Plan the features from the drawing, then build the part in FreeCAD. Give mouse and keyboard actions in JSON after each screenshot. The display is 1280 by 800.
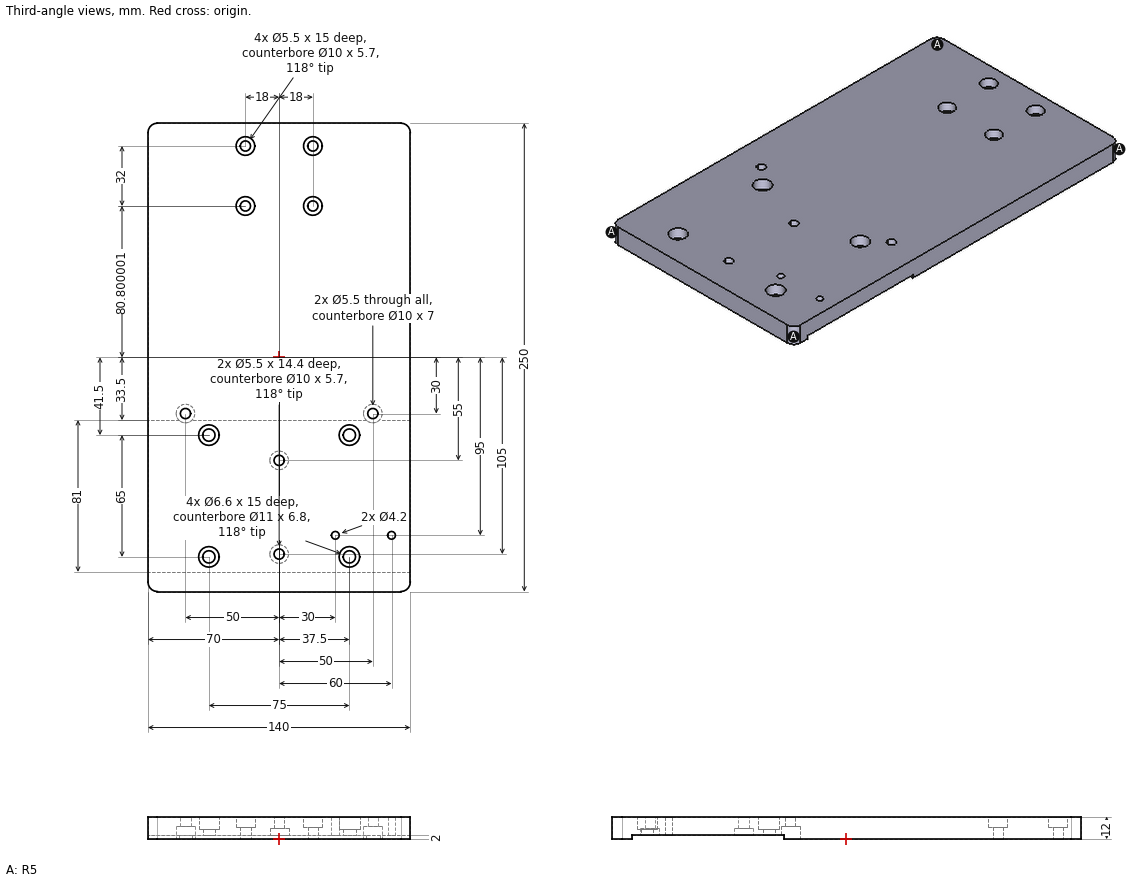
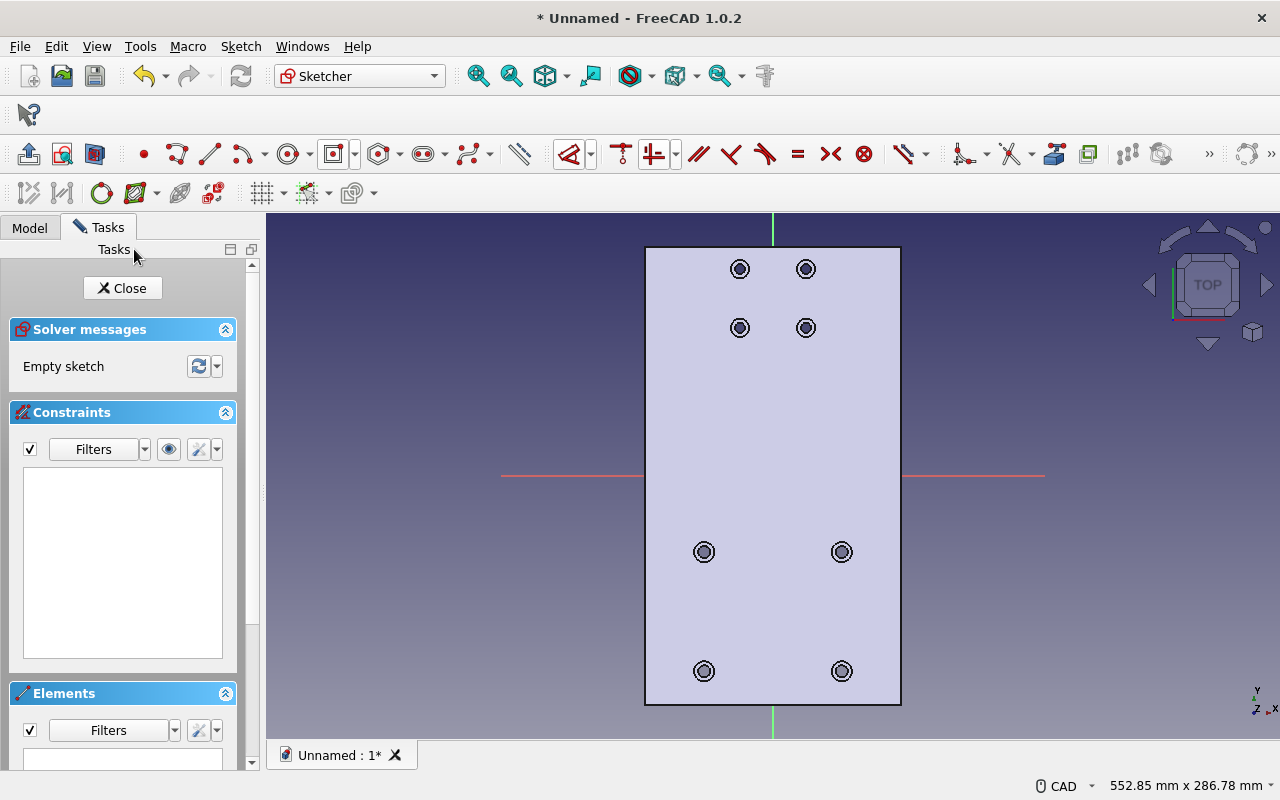
{"action": "left_click", "coordinate": [95, 154]}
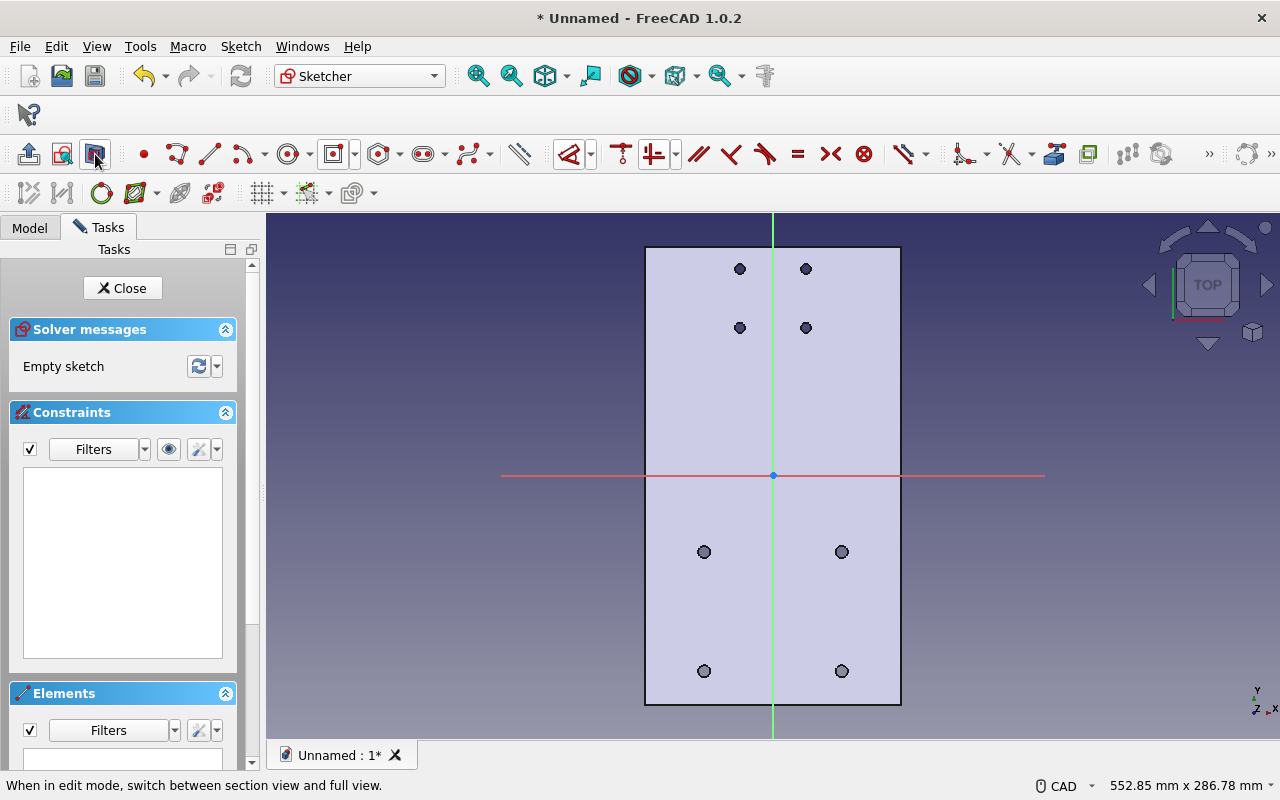
{"action": "scroll", "coordinate": [856, 695], "scroll_direction": "up", "scroll_amount": 3}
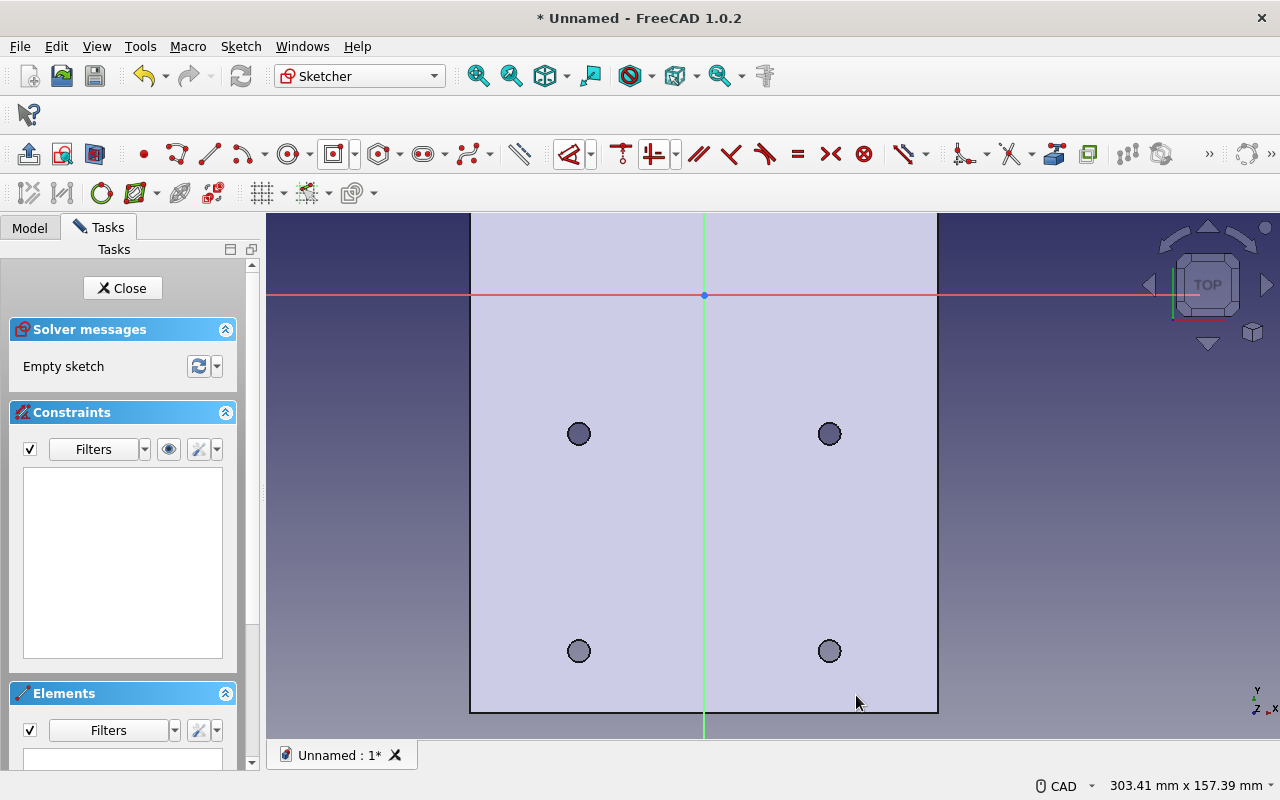
{"action": "left_click", "coordinate": [288, 154]}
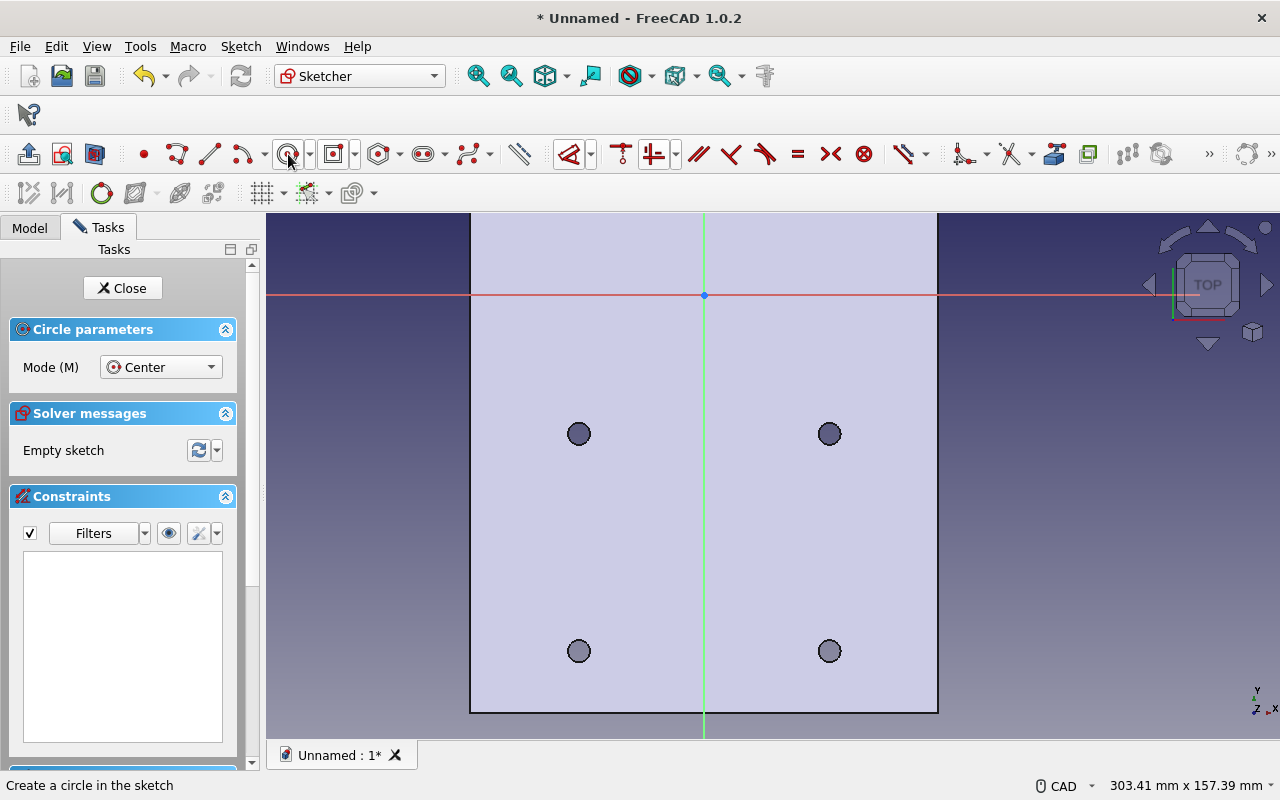
{"action": "scroll", "coordinate": [704, 646], "scroll_direction": "up", "scroll_amount": 5}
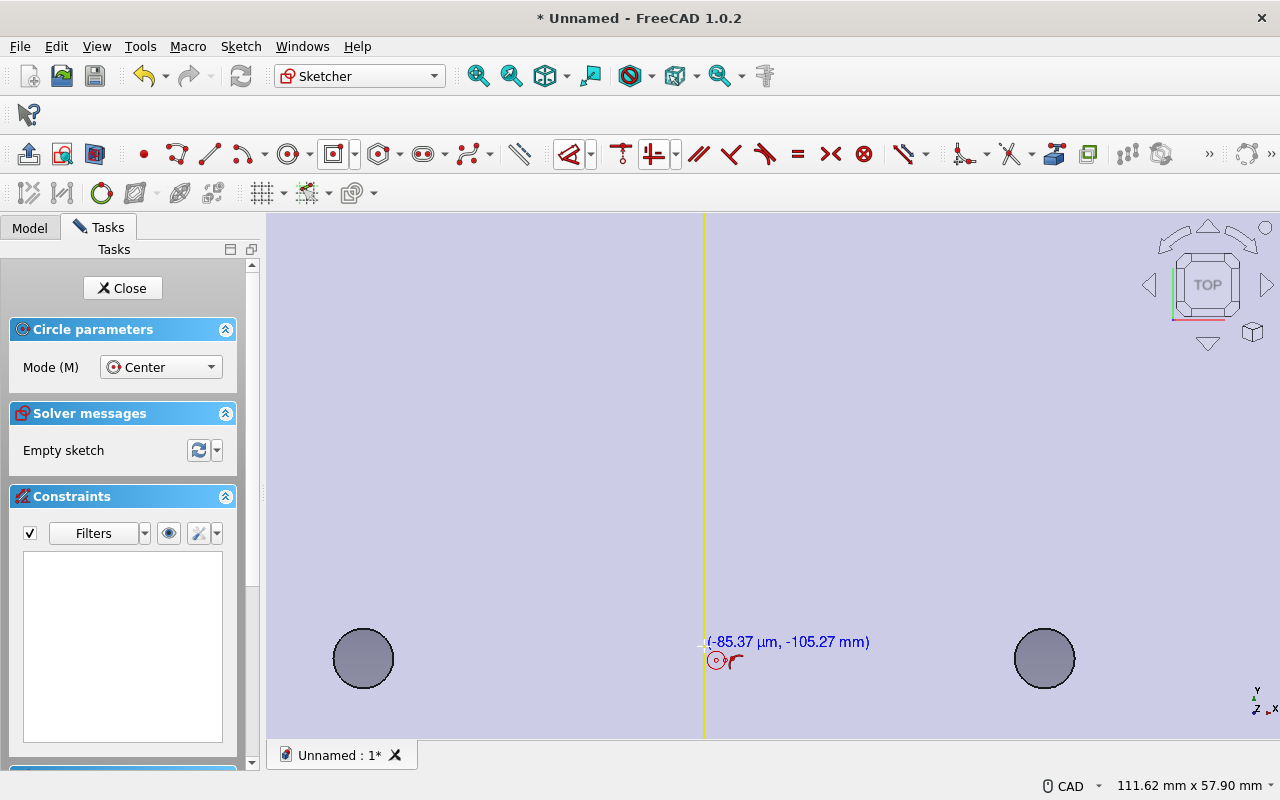
{"action": "left_click", "coordinate": [704, 645]}
{"action": "left_click", "coordinate": [722, 627]}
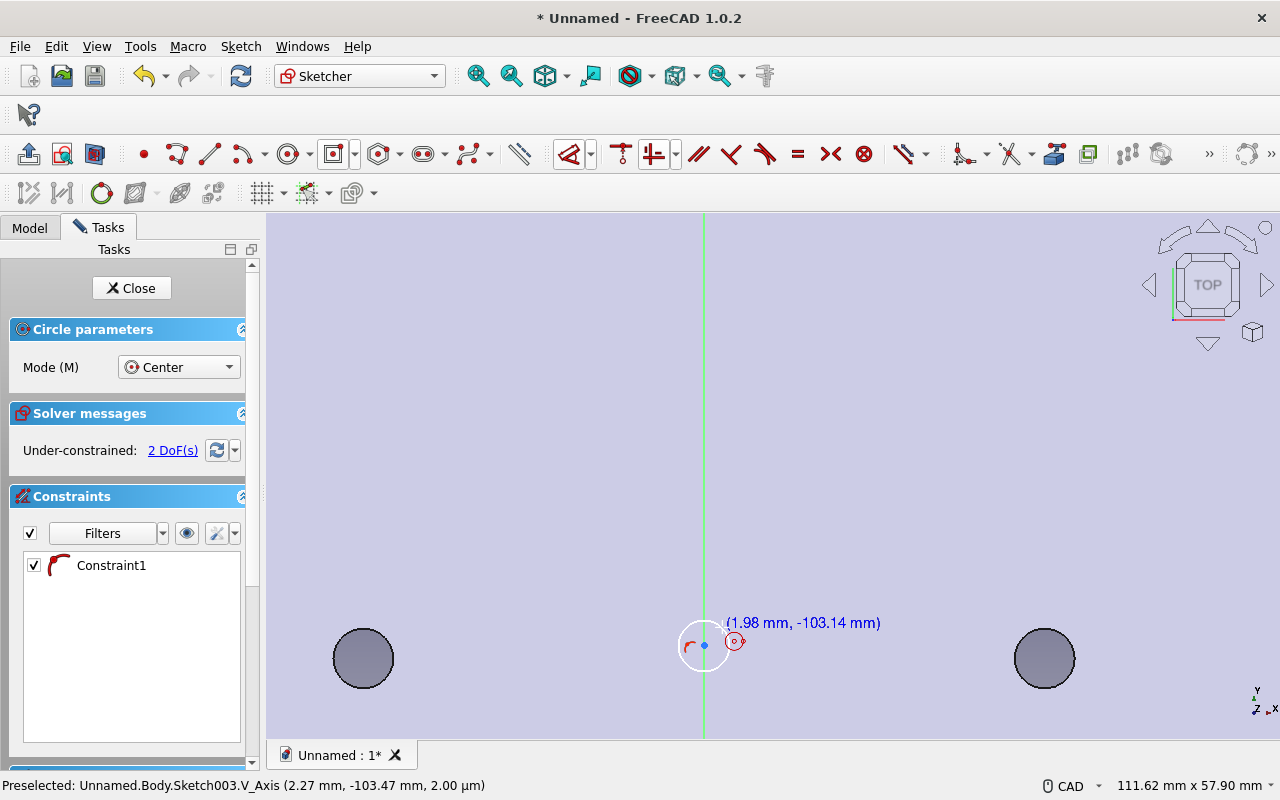
{"action": "scroll", "coordinate": [705, 648], "scroll_direction": "down", "scroll_amount": 5}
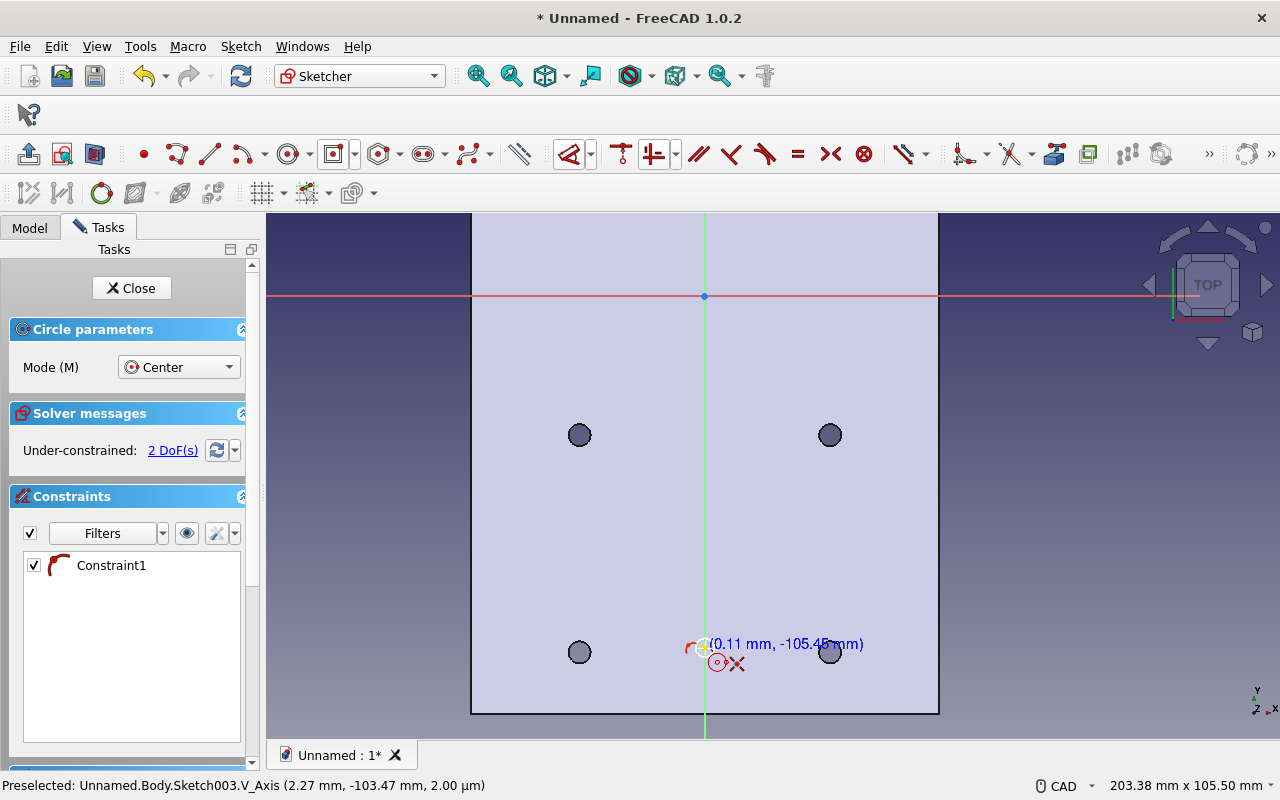
{"action": "scroll", "coordinate": [705, 480], "scroll_direction": "up", "scroll_amount": 5}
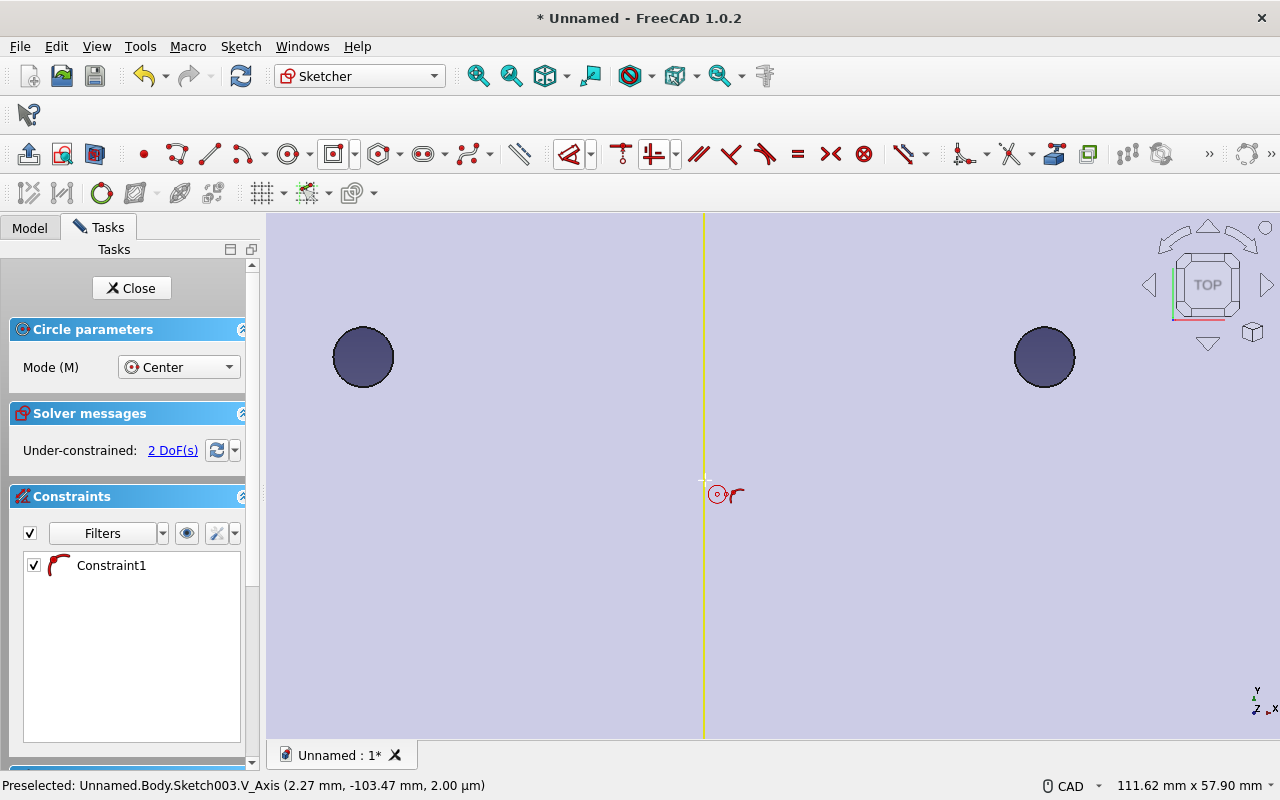
{"action": "left_click", "coordinate": [704, 480]}
{"action": "left_click", "coordinate": [722, 462]}
{"action": "key", "text": "Escape"}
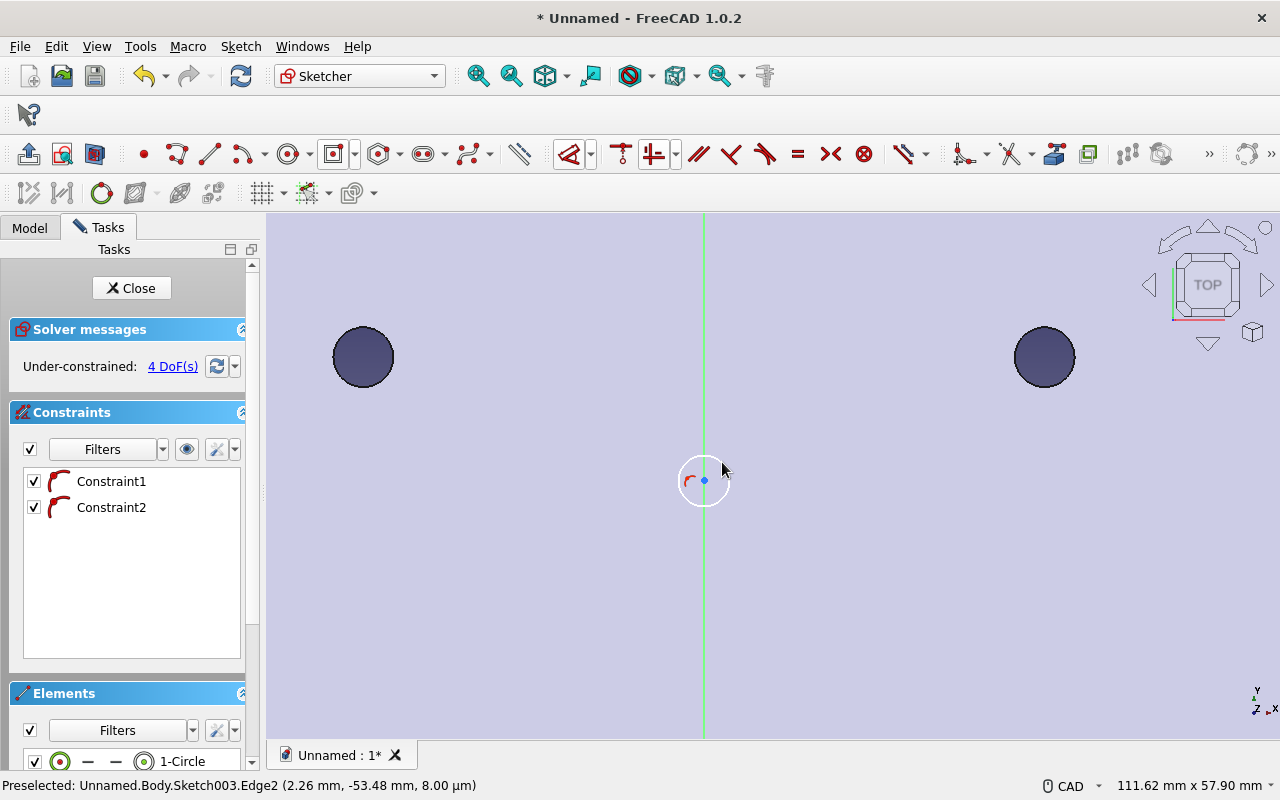
{"action": "scroll", "coordinate": [705, 480], "scroll_direction": "down", "scroll_amount": 5}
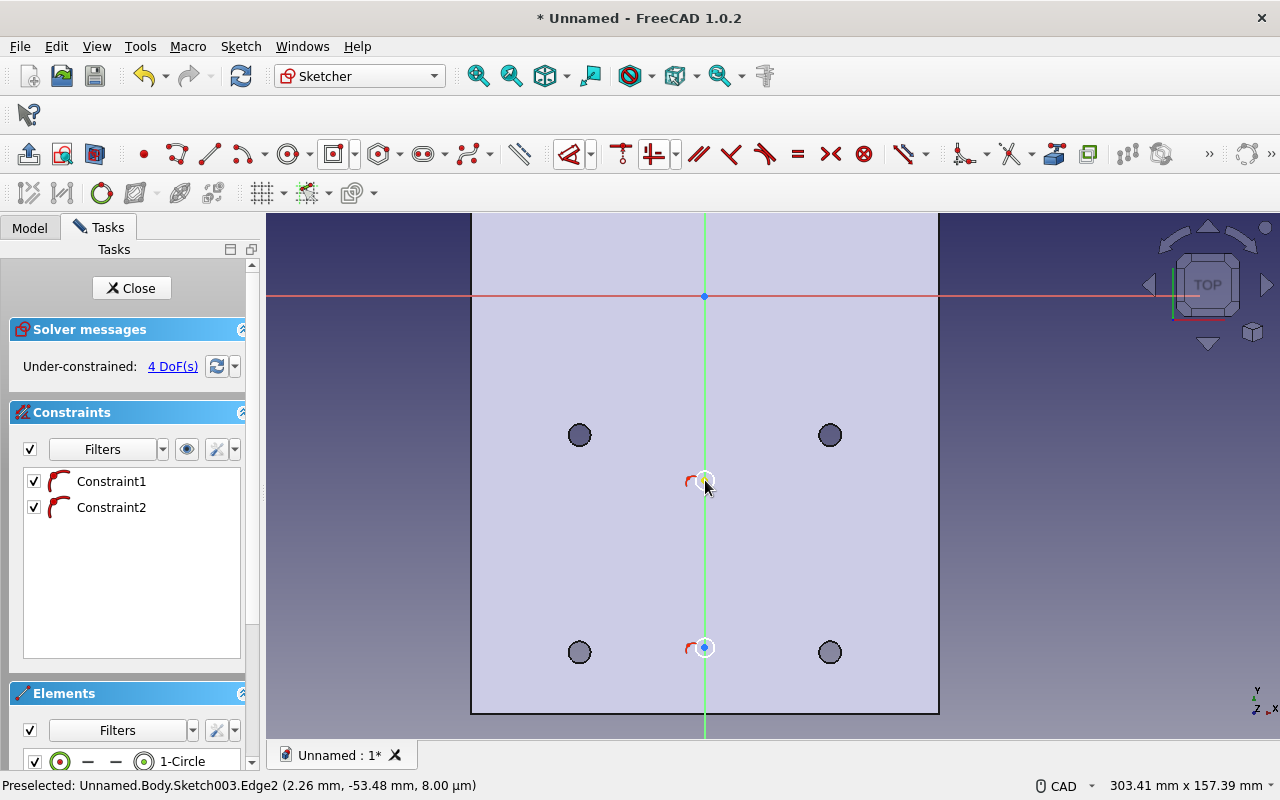
{"action": "scroll", "coordinate": [712, 641], "scroll_direction": "up", "scroll_amount": 4}